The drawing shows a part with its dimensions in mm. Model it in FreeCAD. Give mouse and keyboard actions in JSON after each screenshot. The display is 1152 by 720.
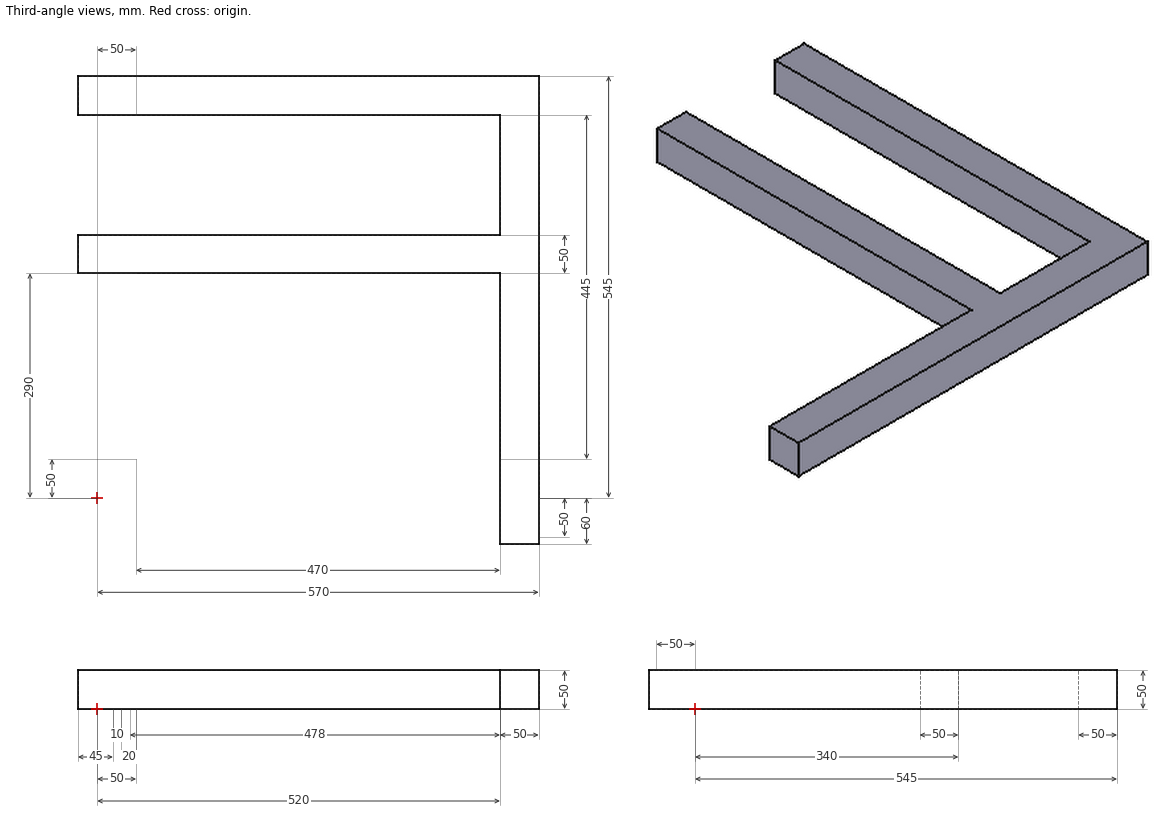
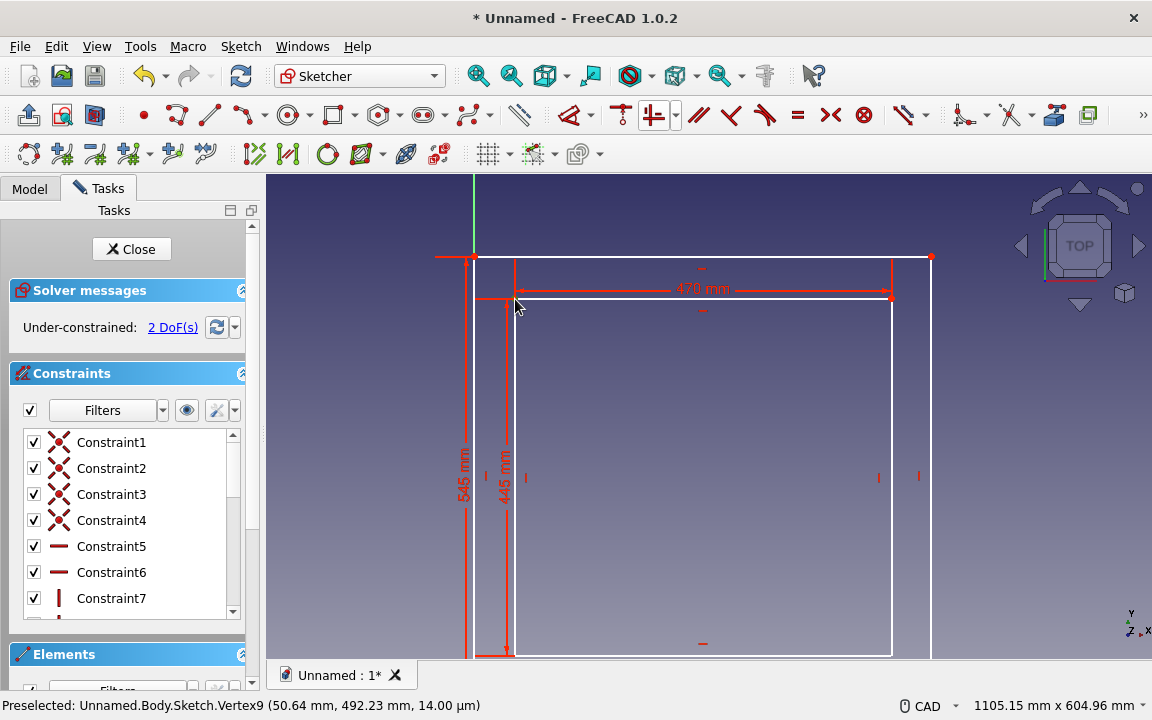
{"action": "key", "text": "l"}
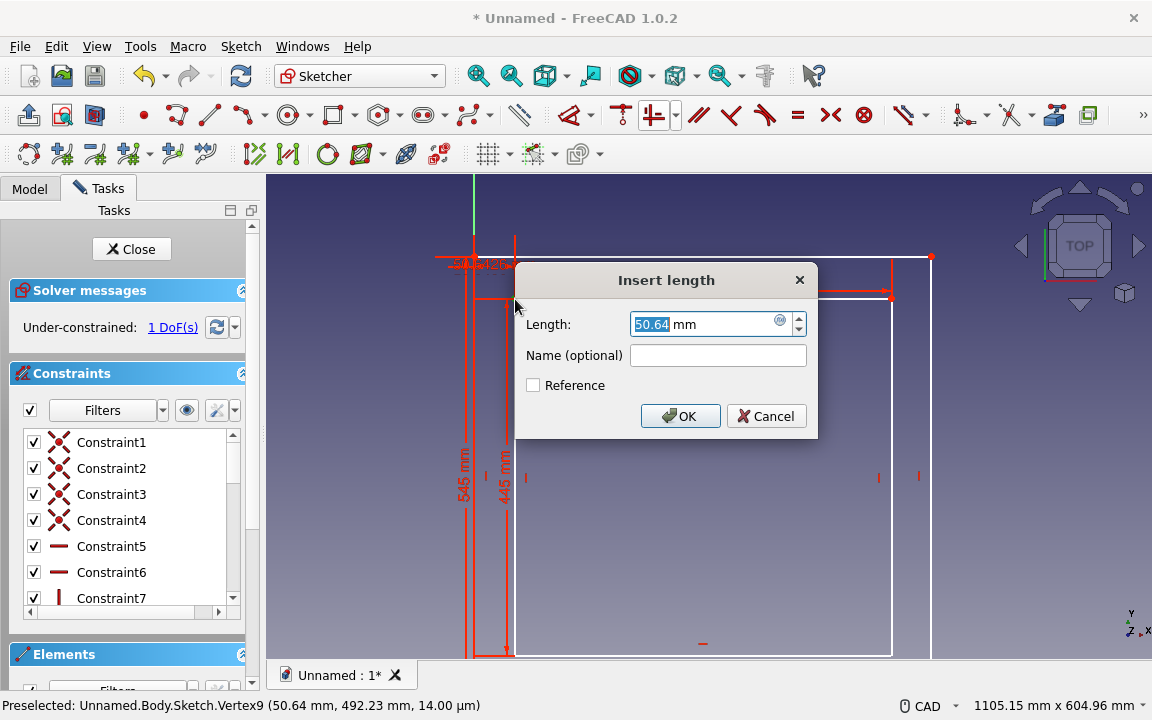
{"action": "type", "text": "50"}
{"action": "key", "text": "Return"}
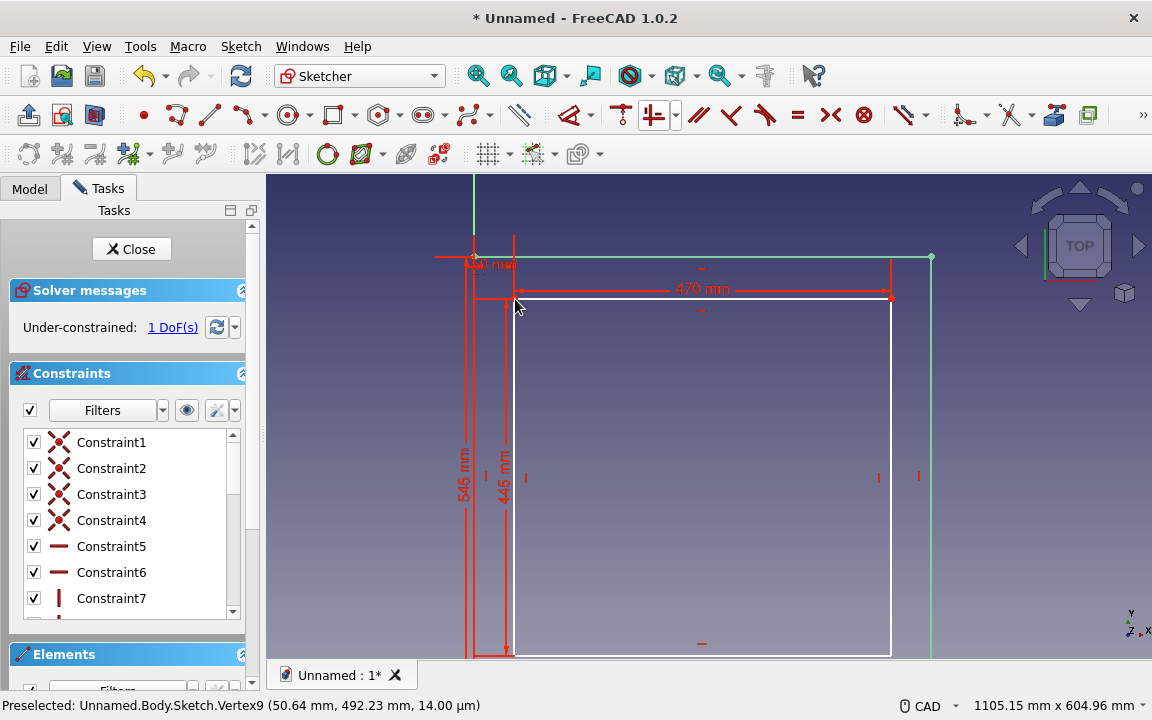
{"action": "scroll", "coordinate": [514, 297], "scroll_direction": "down", "scroll_amount": 2}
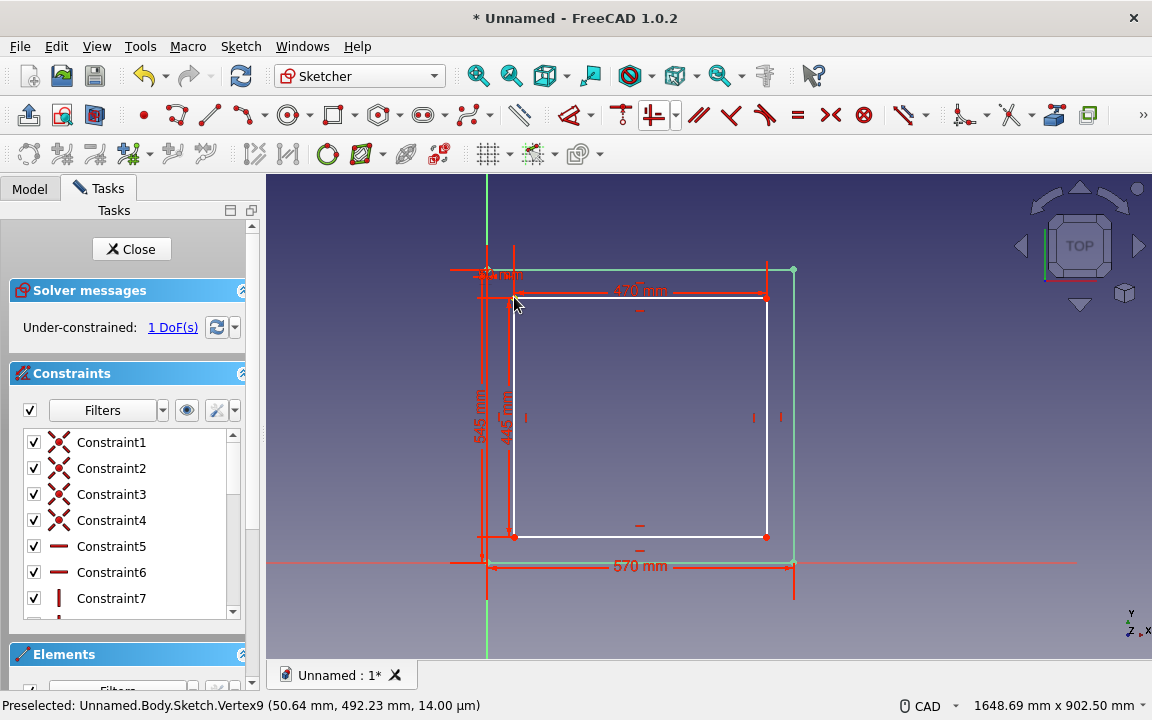
{"action": "scroll", "coordinate": [514, 537], "scroll_direction": "up", "scroll_amount": 2}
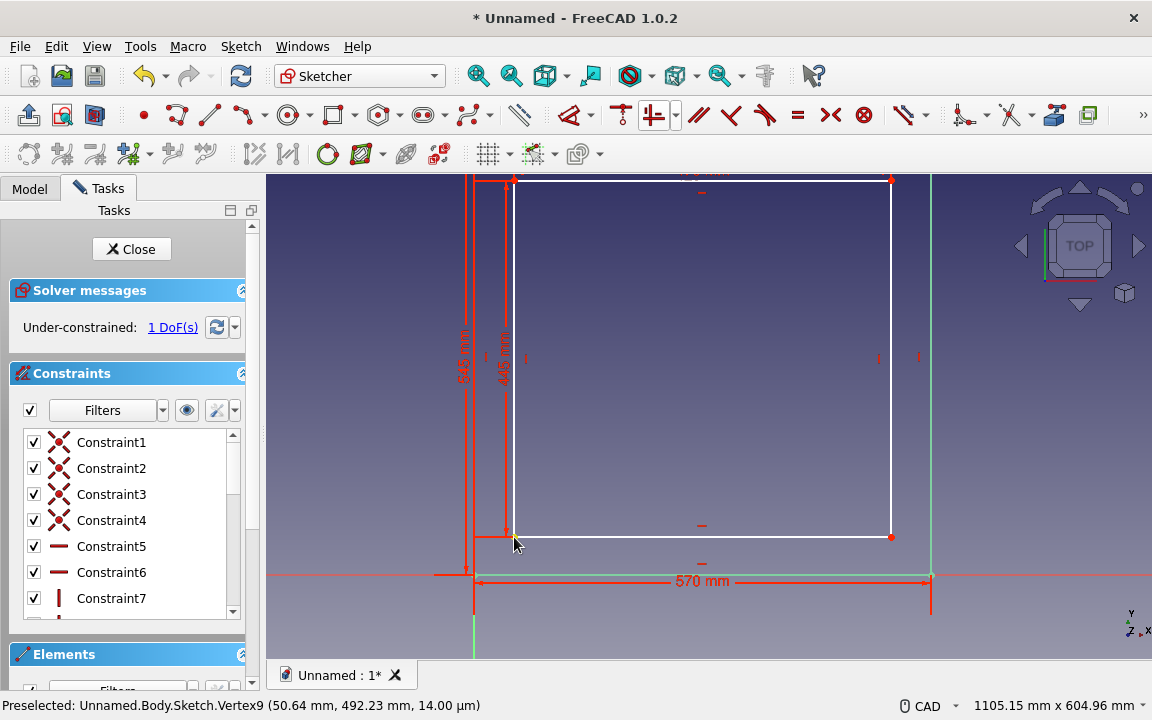
{"action": "left_click", "coordinate": [514, 537]}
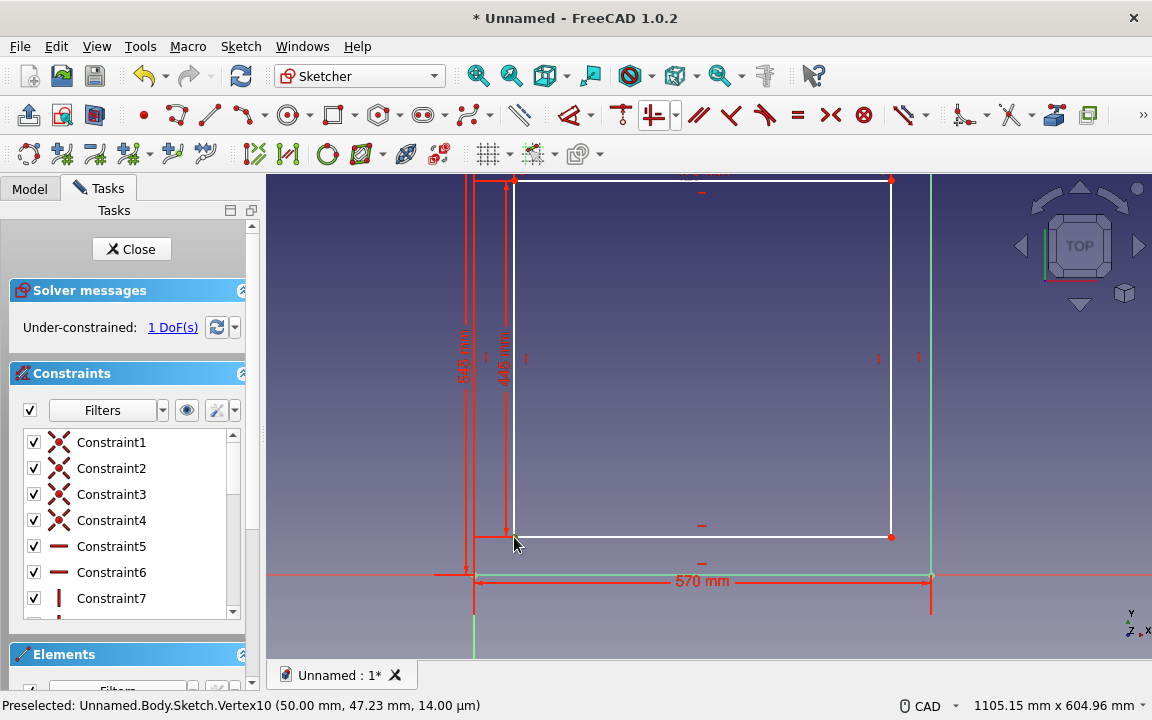
{"action": "left_click", "coordinate": [590, 116]}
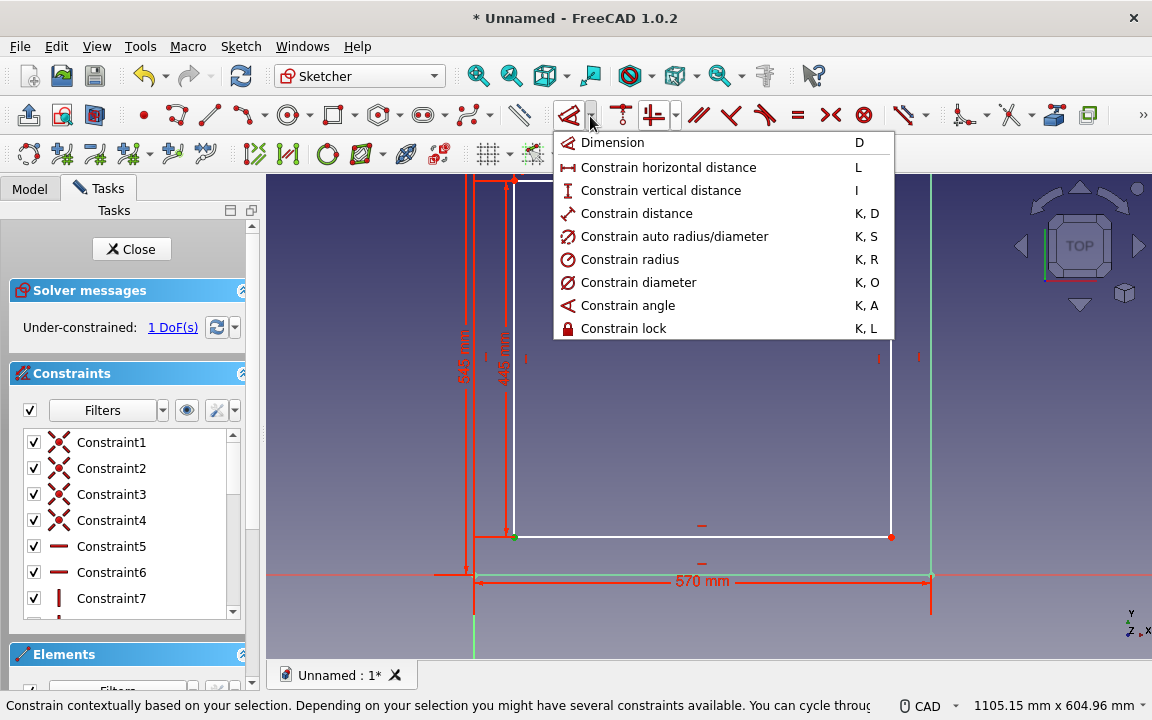
{"action": "left_click", "coordinate": [724, 190]}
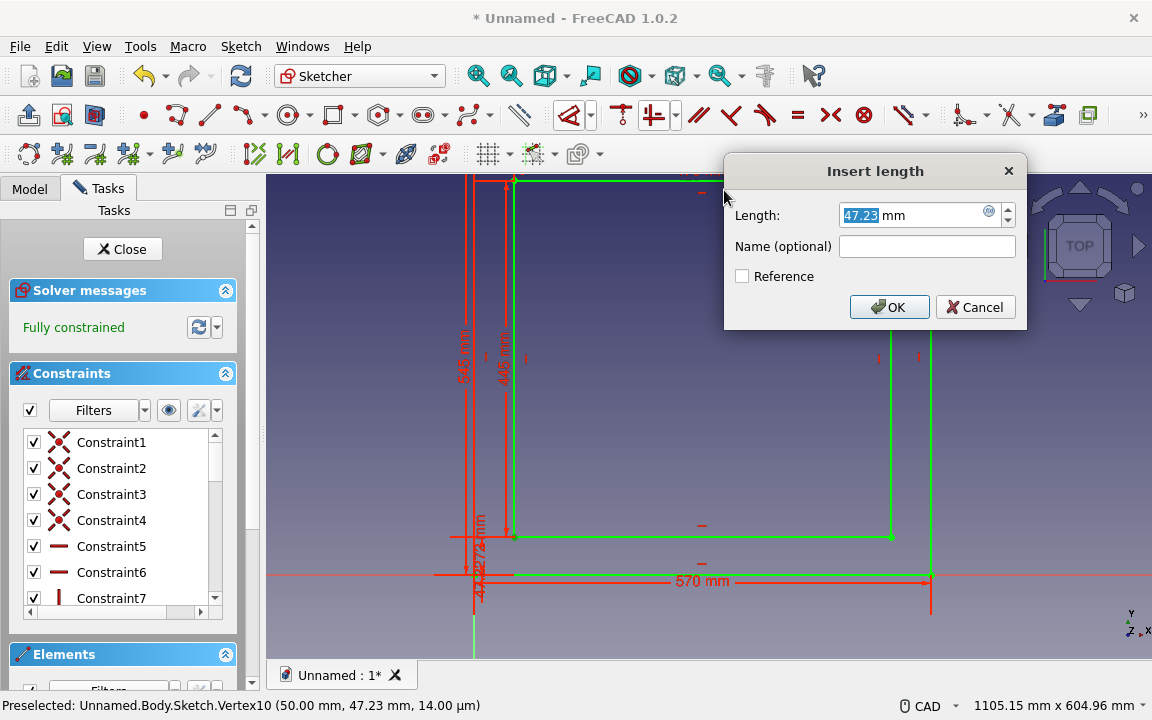
{"action": "type", "text": "50"}
{"action": "key", "text": "Return"}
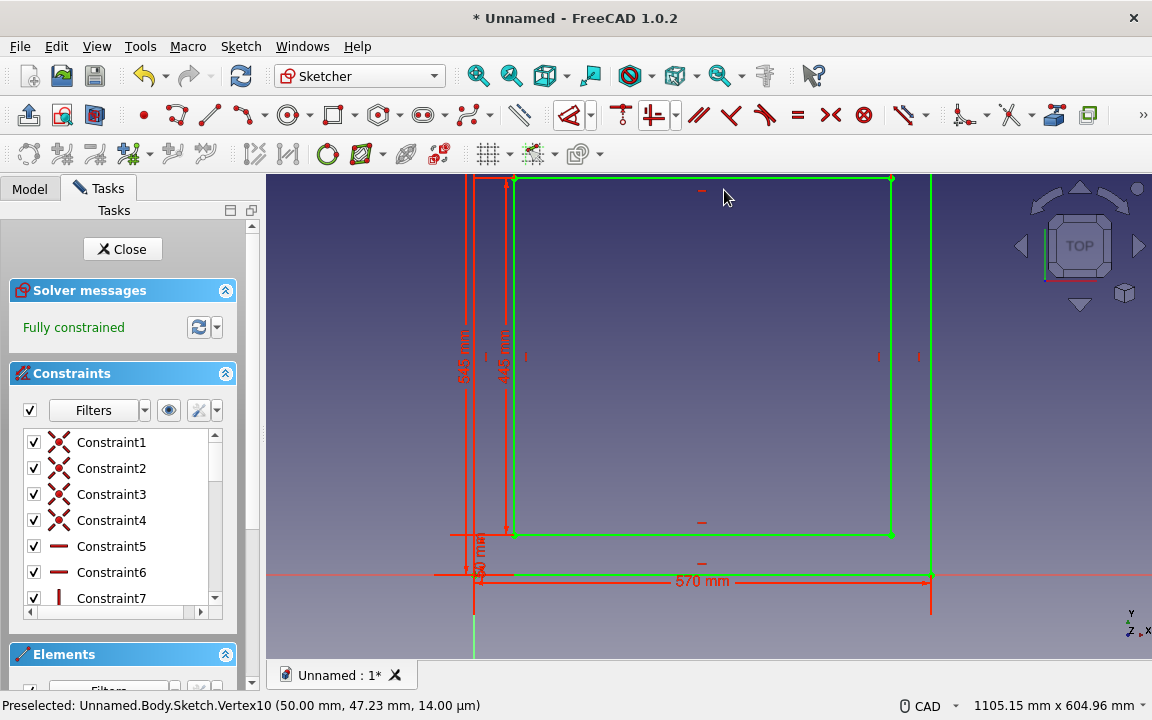
{"action": "left_click", "coordinate": [123, 249]}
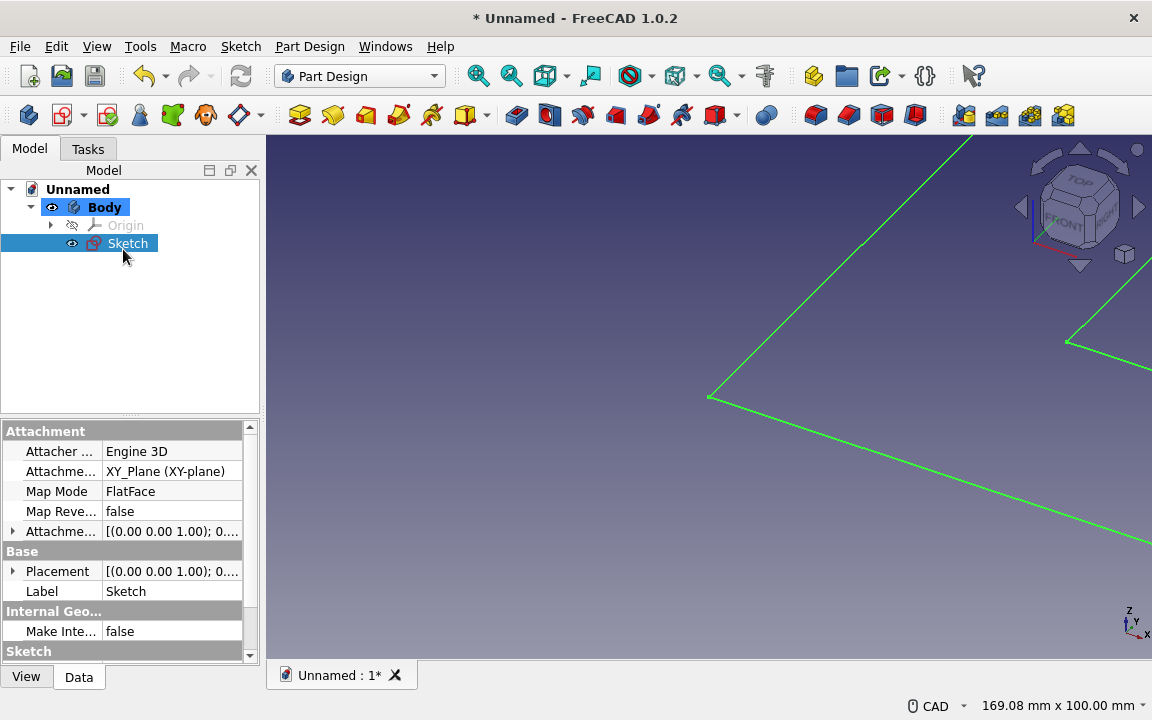
{"action": "left_click", "coordinate": [300, 116]}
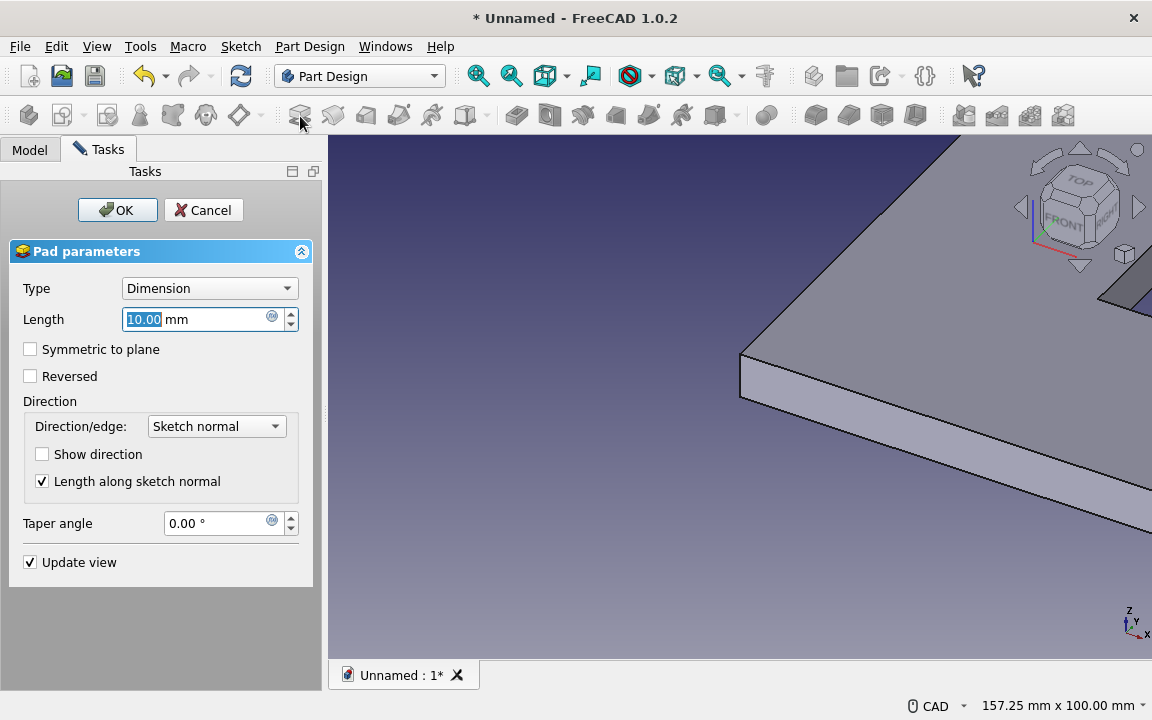
{"action": "type", "text": "50"}
{"action": "key", "text": "Tab"}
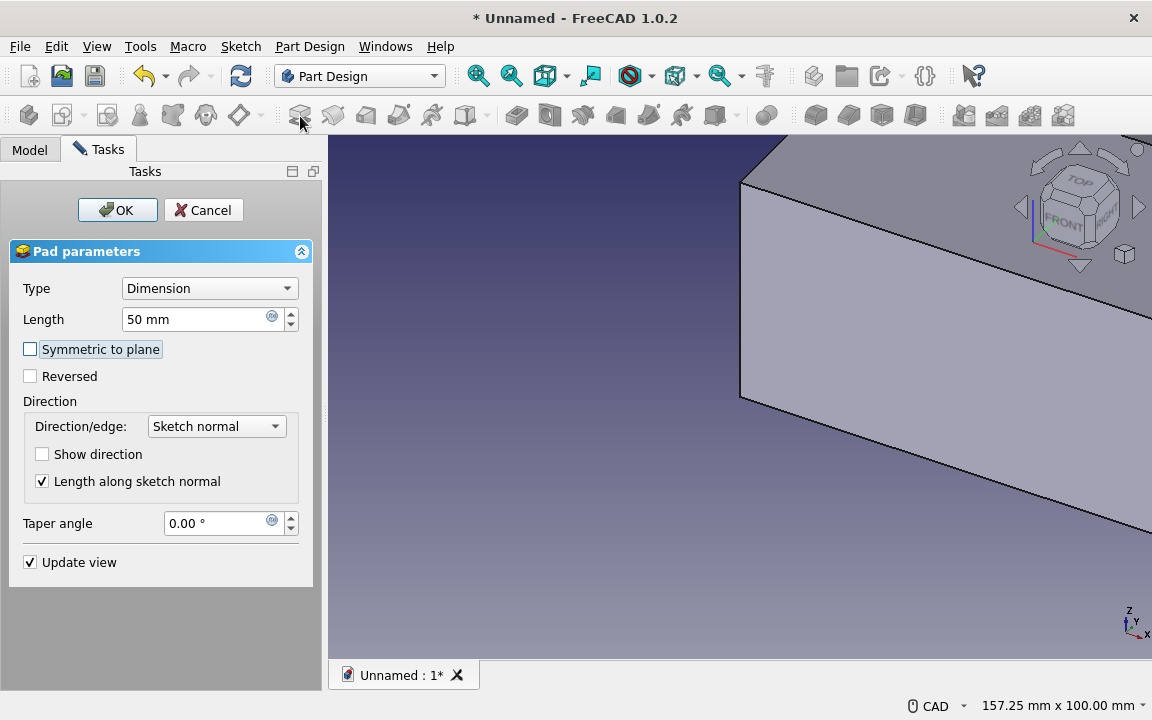
{"action": "left_click", "coordinate": [118, 210]}